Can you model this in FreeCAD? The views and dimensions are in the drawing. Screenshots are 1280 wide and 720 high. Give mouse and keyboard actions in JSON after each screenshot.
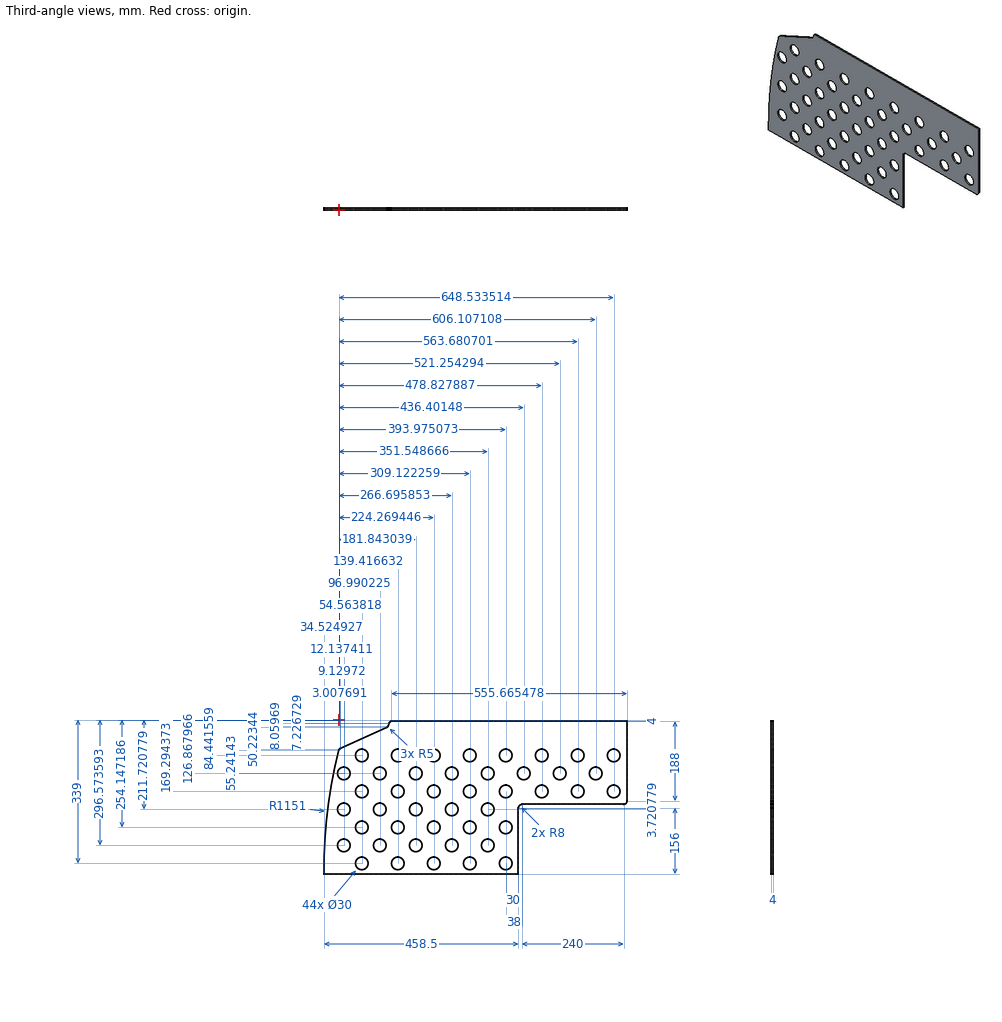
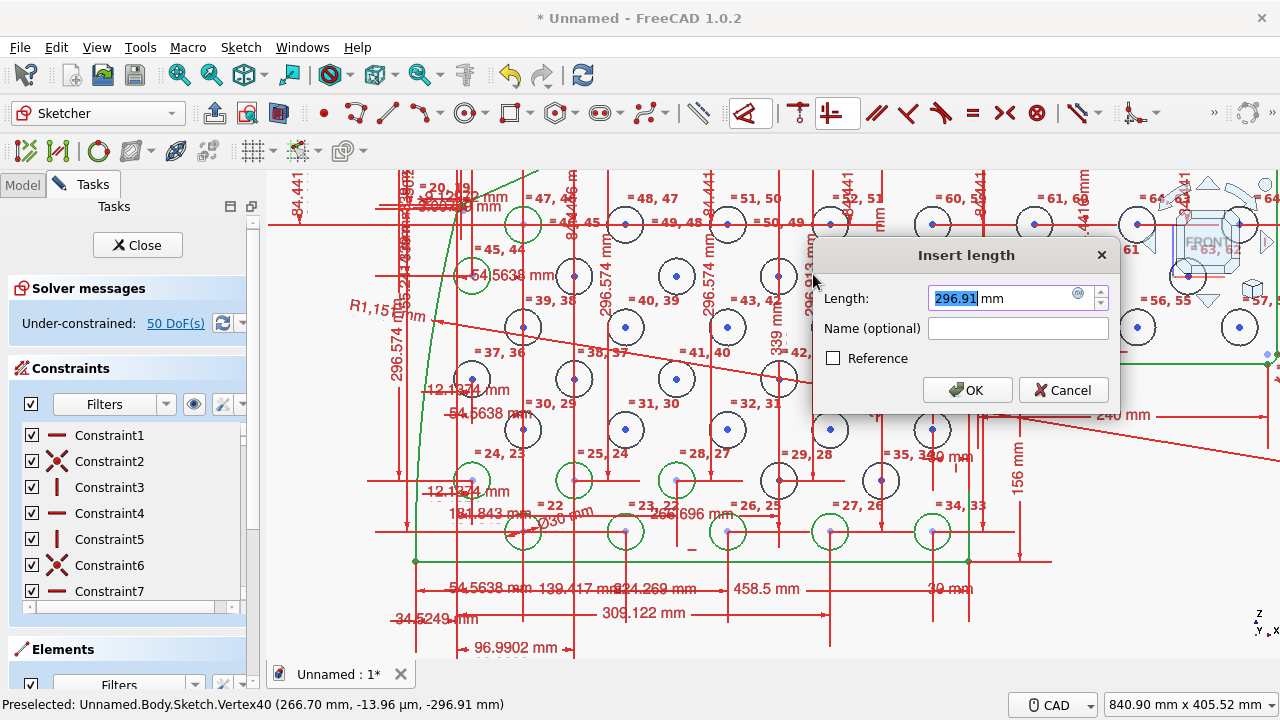
{"action": "type", "text": "296.573593"}
{"action": "key", "text": "Return"}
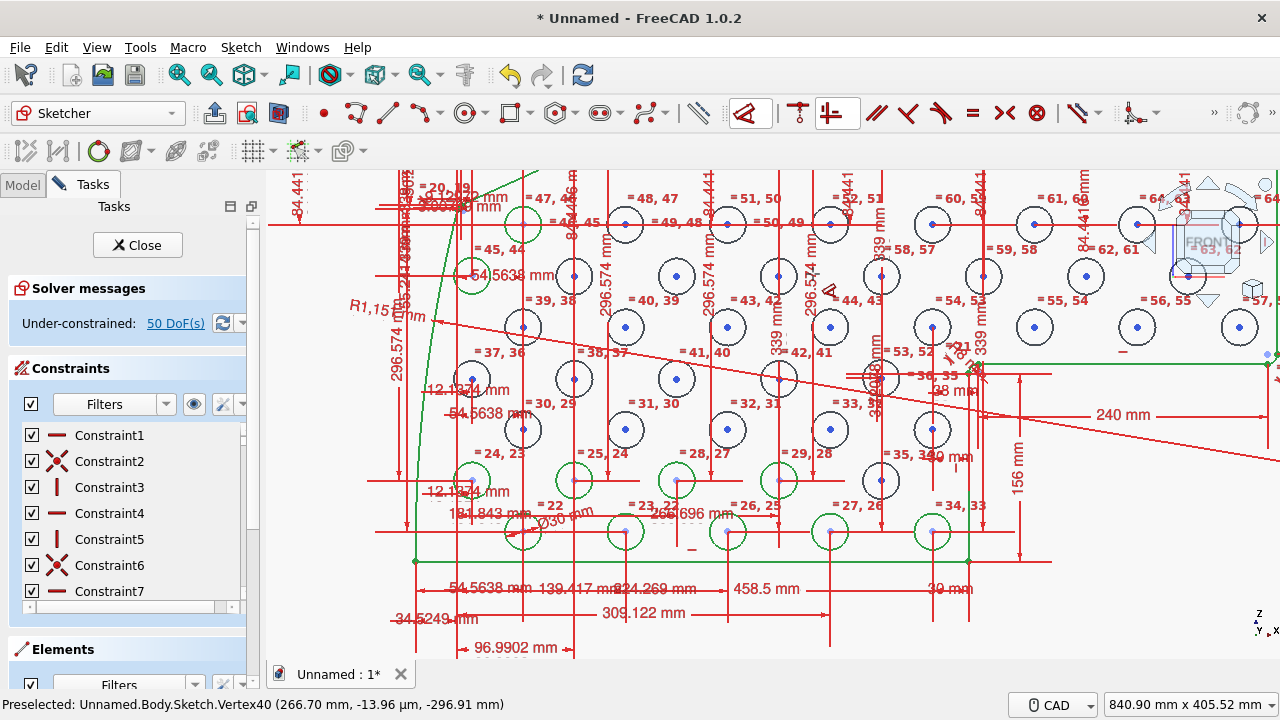
{"action": "left_click", "coordinate": [523, 430]}
{"action": "left_click", "coordinate": [557, 314]}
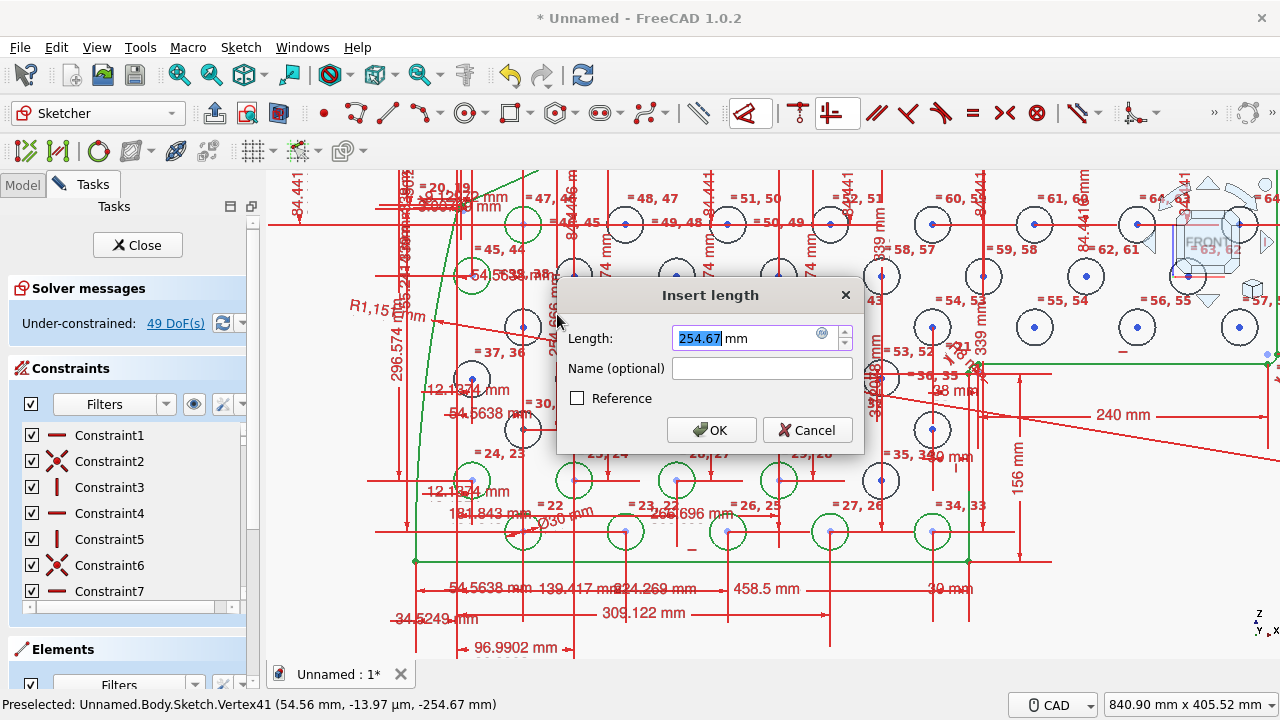
{"action": "type", "text": "254.147186"}
{"action": "key", "text": "Return"}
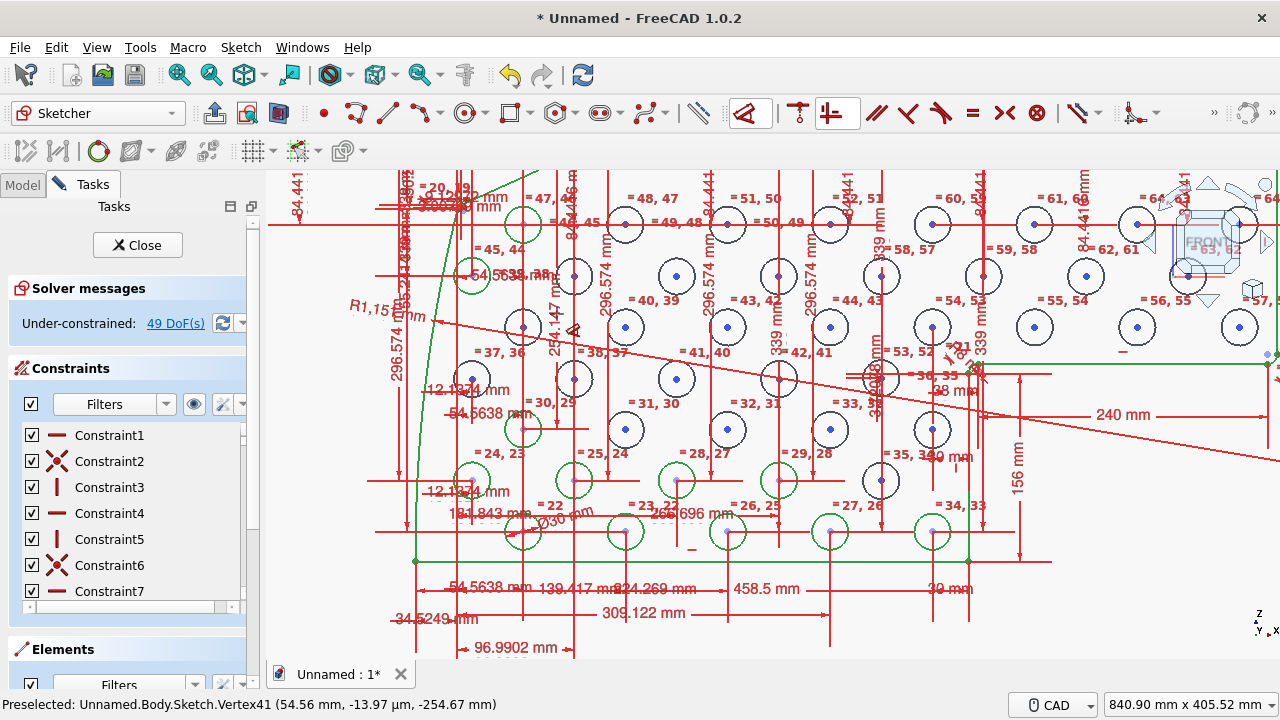
{"action": "left_click", "coordinate": [626, 430]}
{"action": "left_click", "coordinate": [542, 464]}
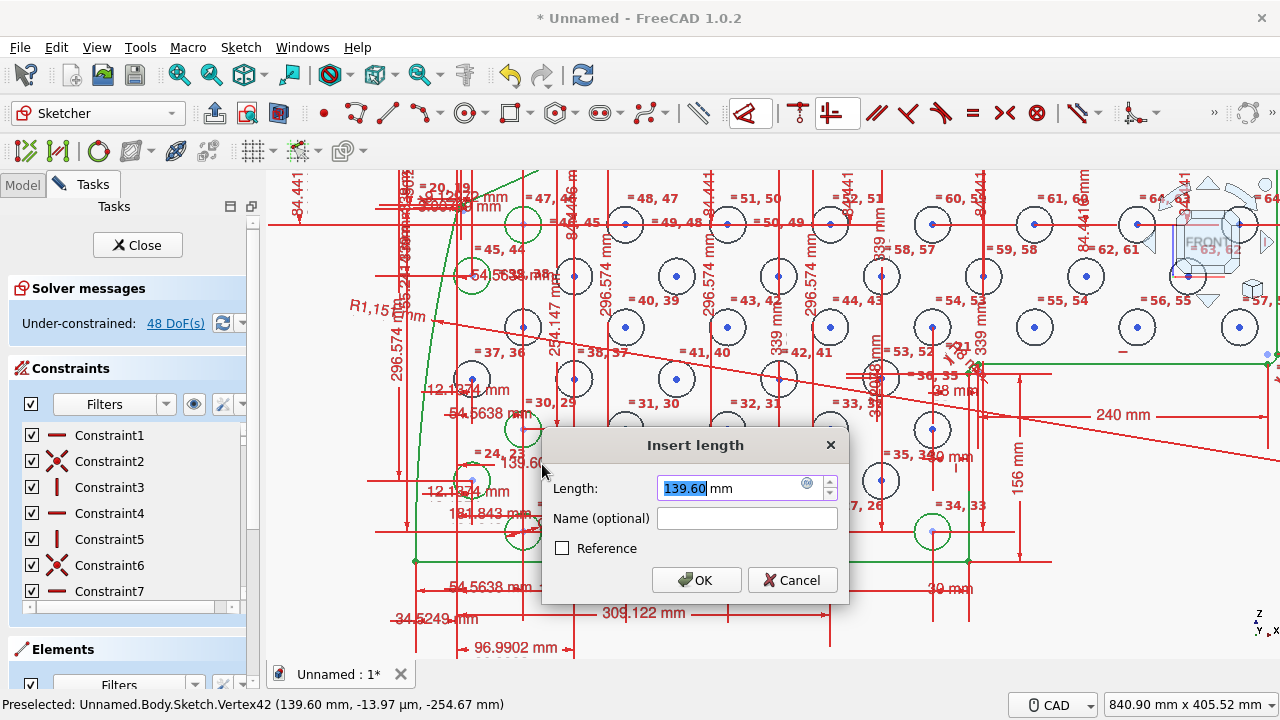
{"action": "type", "text": "139.416632"}
{"action": "key", "text": "Return"}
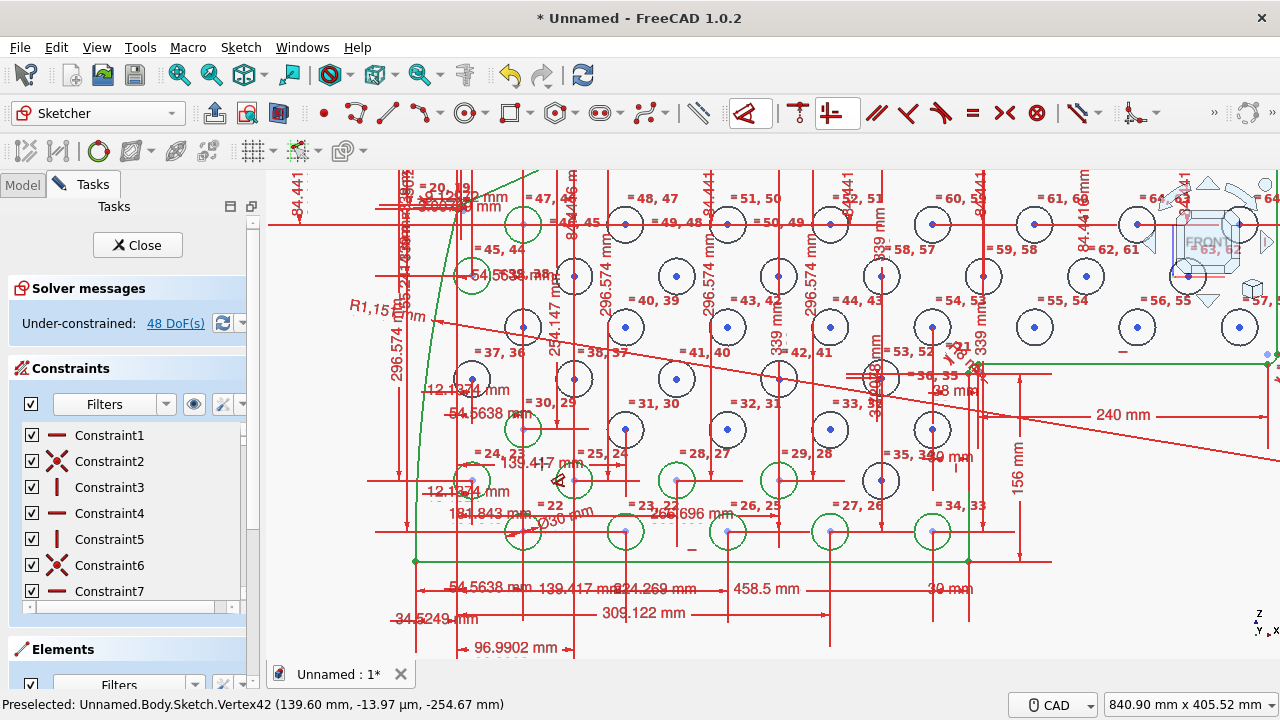
{"action": "left_click", "coordinate": [626, 430]}
{"action": "left_click", "coordinate": [660, 314]}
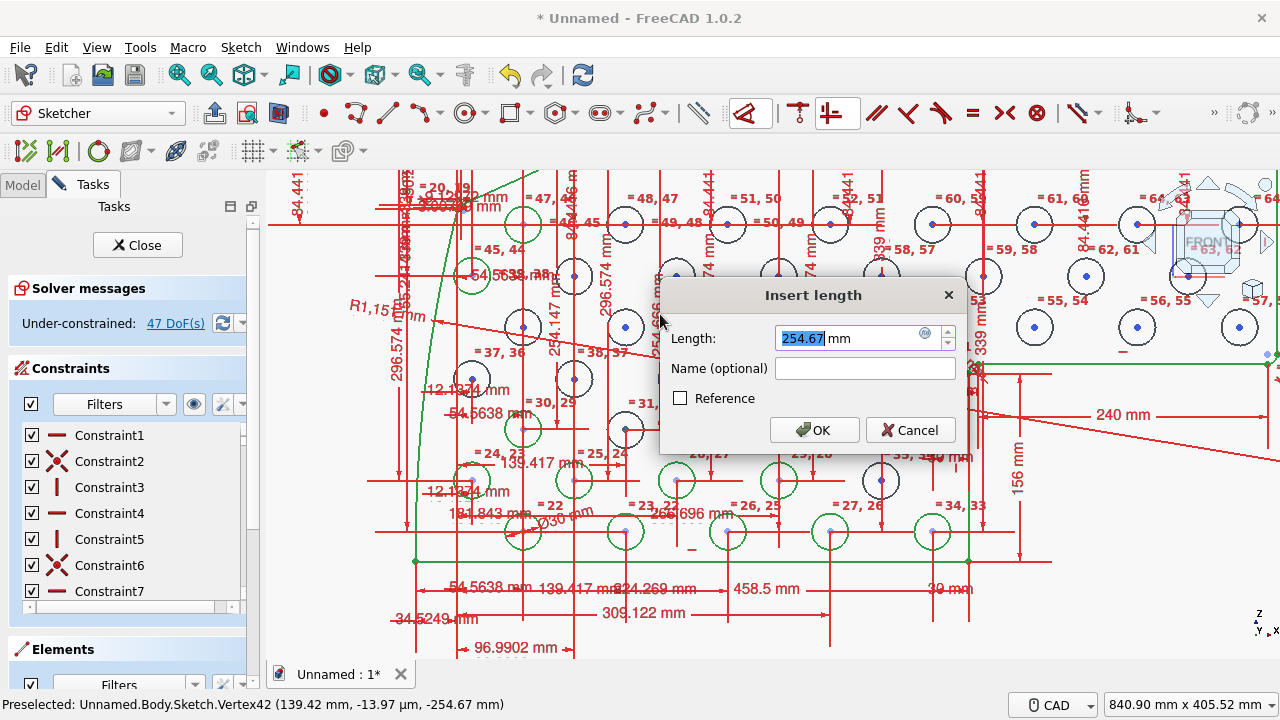
{"action": "type", "text": "254.147186"}
{"action": "key", "text": "Return"}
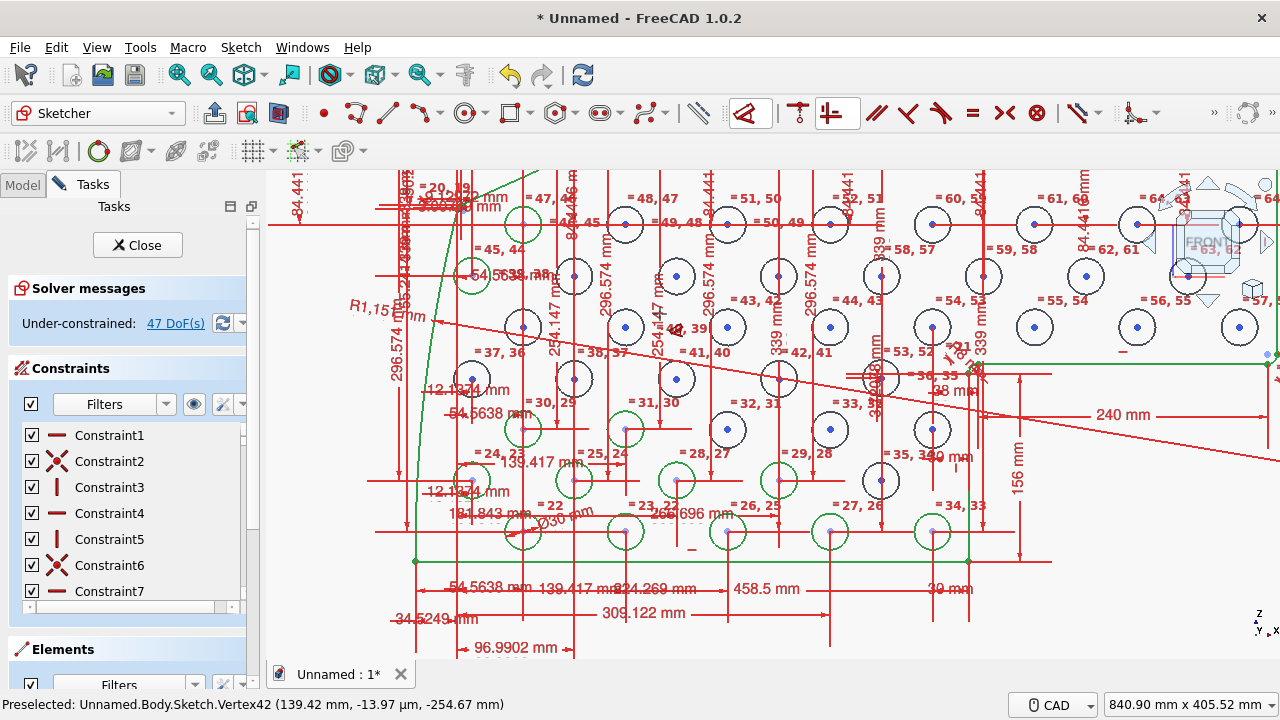
{"action": "left_click", "coordinate": [728, 430]}
{"action": "left_click", "coordinate": [687, 536]}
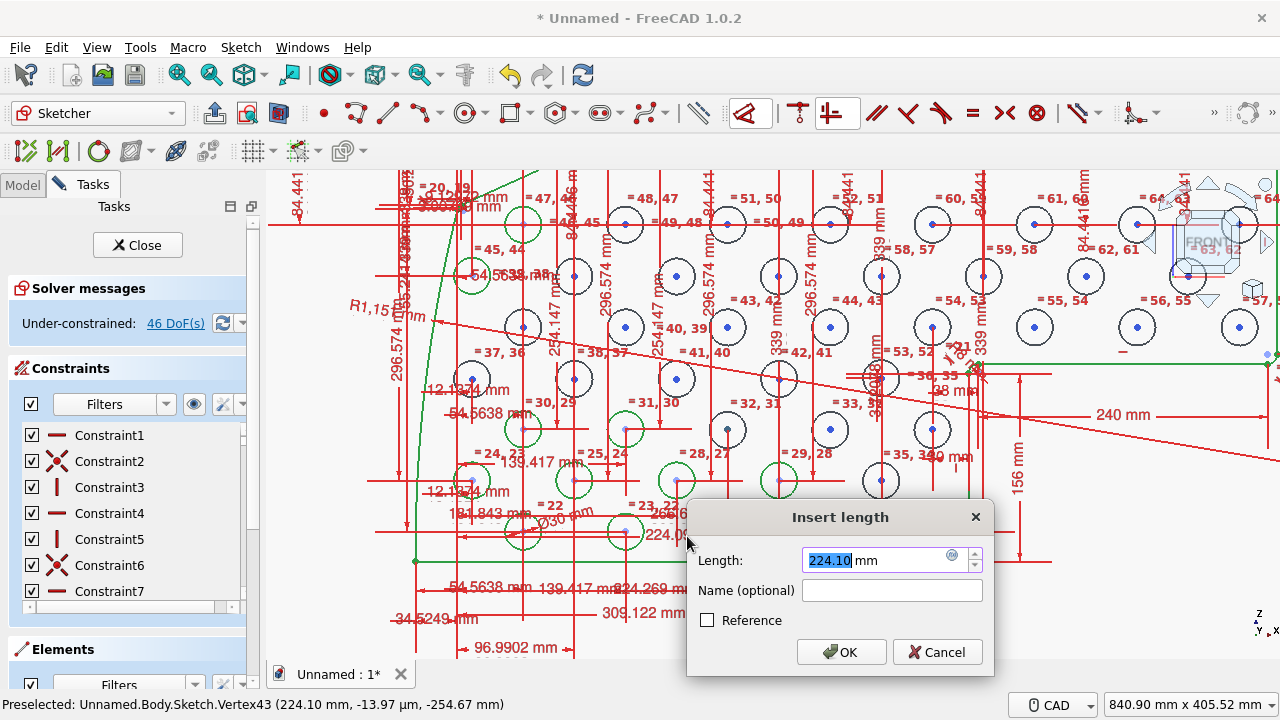
{"action": "type", "text": "224.269446"}
{"action": "key", "text": "Return"}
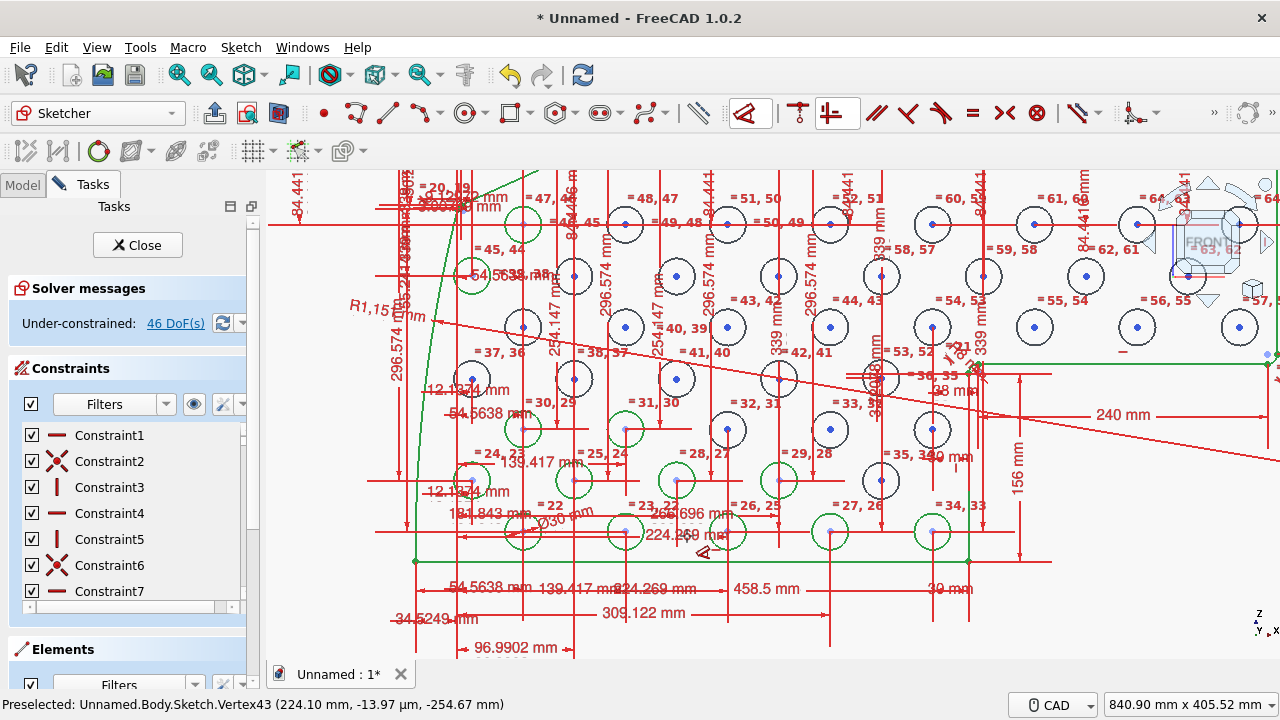
{"action": "left_click", "coordinate": [728, 430]}
{"action": "left_click", "coordinate": [762, 233]}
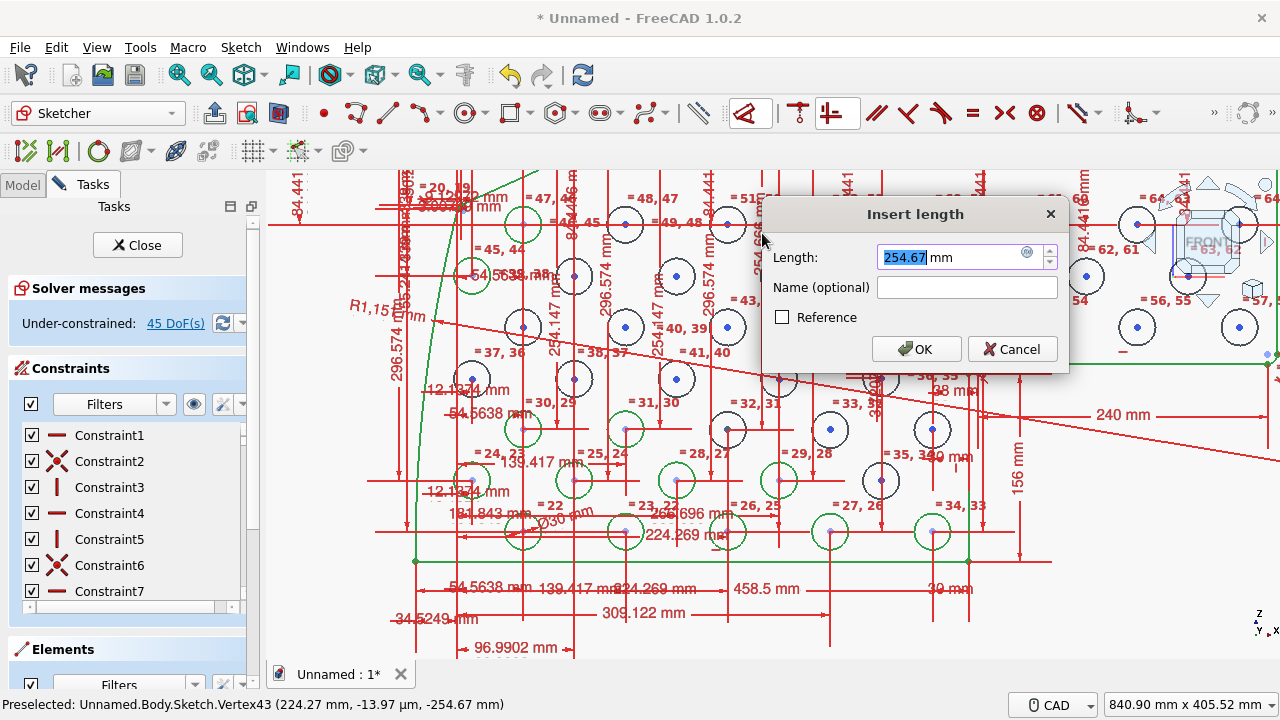
{"action": "type", "text": "254.147186"}
{"action": "key", "text": "Return"}